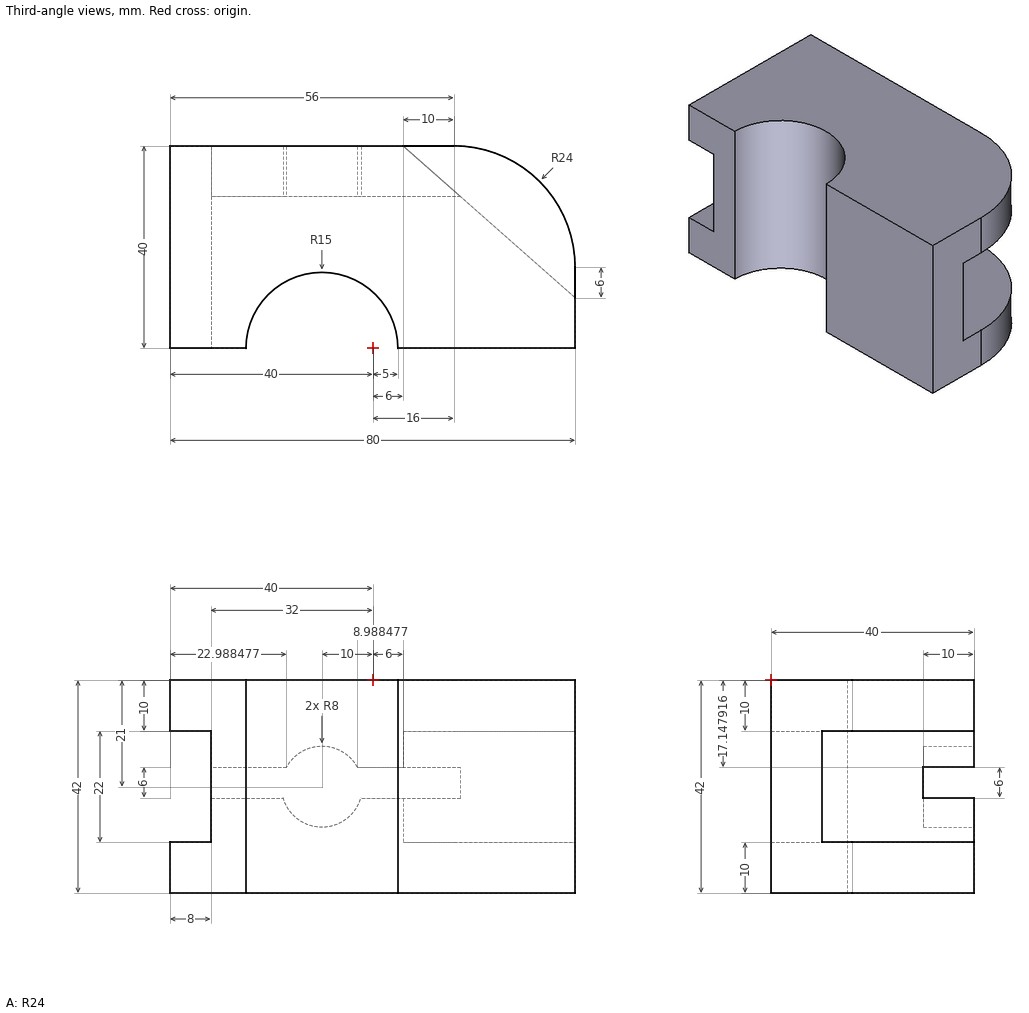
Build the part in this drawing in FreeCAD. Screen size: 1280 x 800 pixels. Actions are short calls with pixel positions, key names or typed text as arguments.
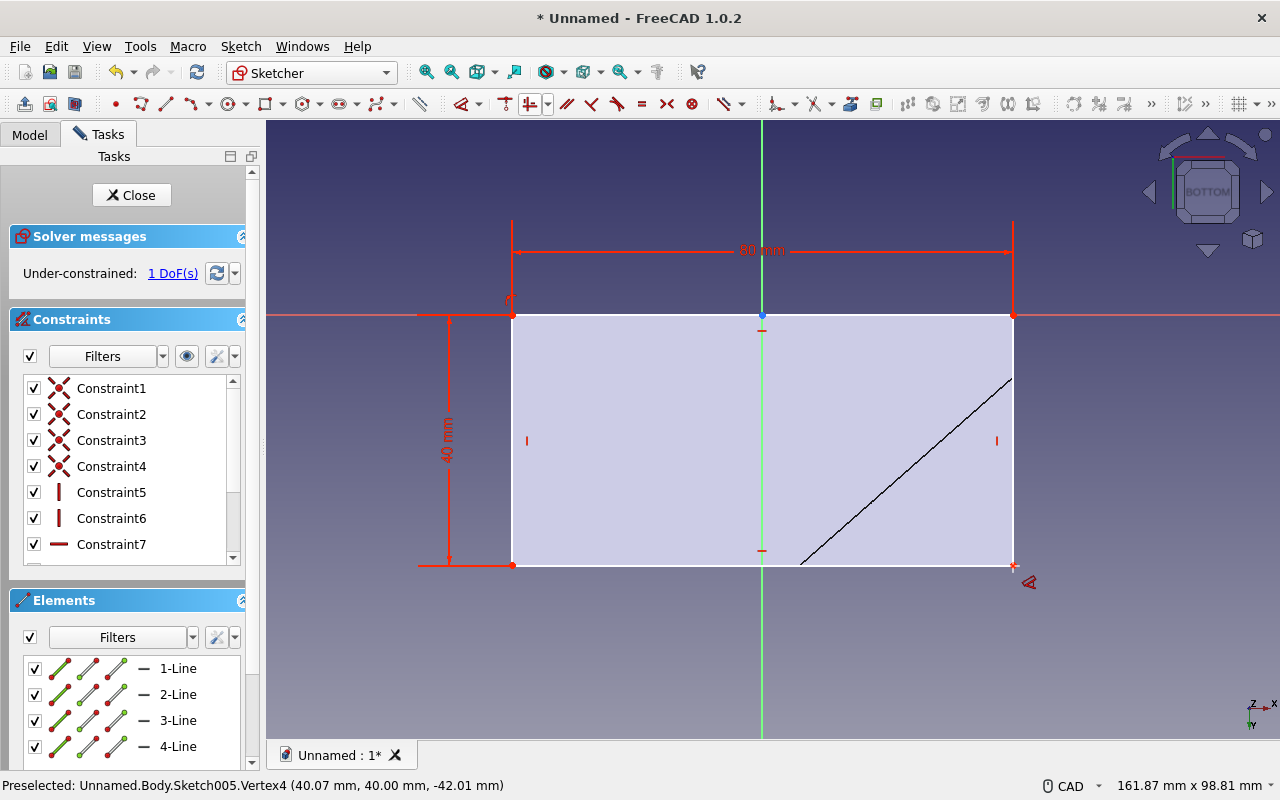
click(512, 315)
click(637, 281)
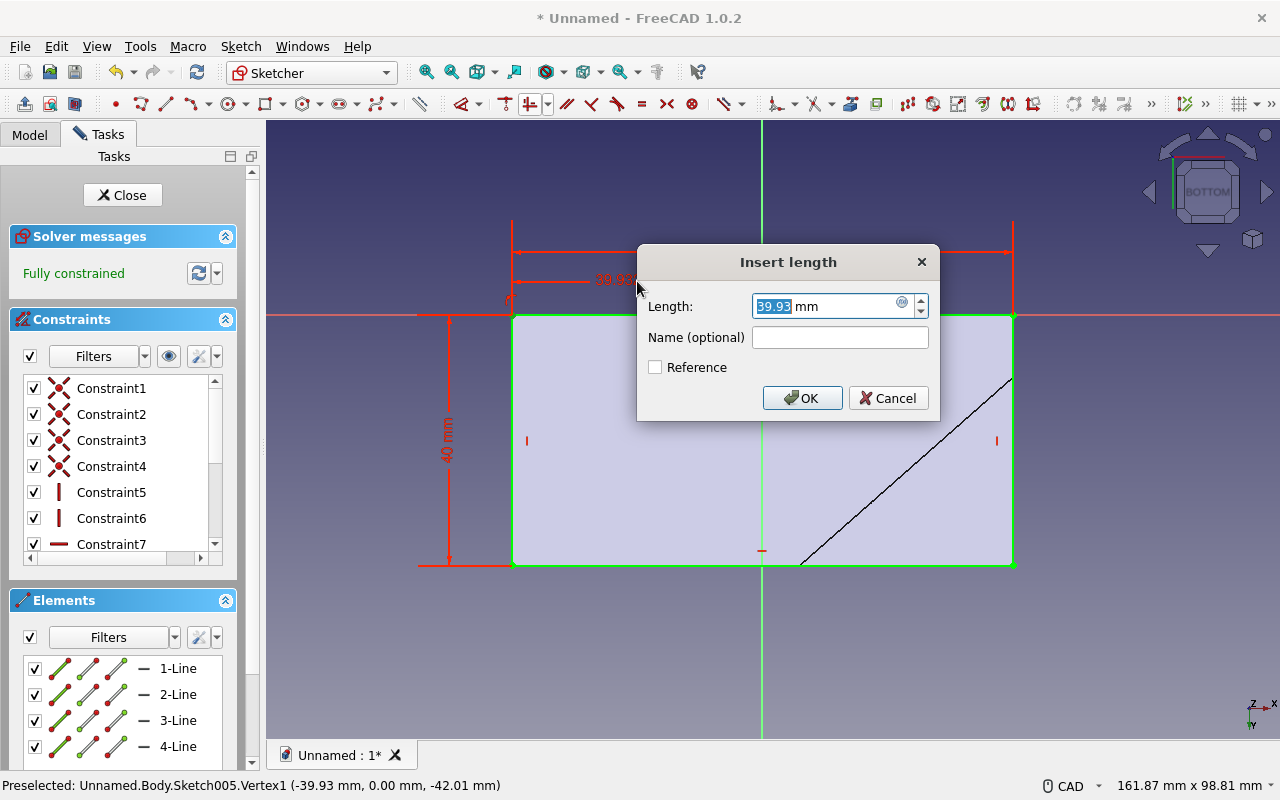
text(40)
key(Return)
key(Escape)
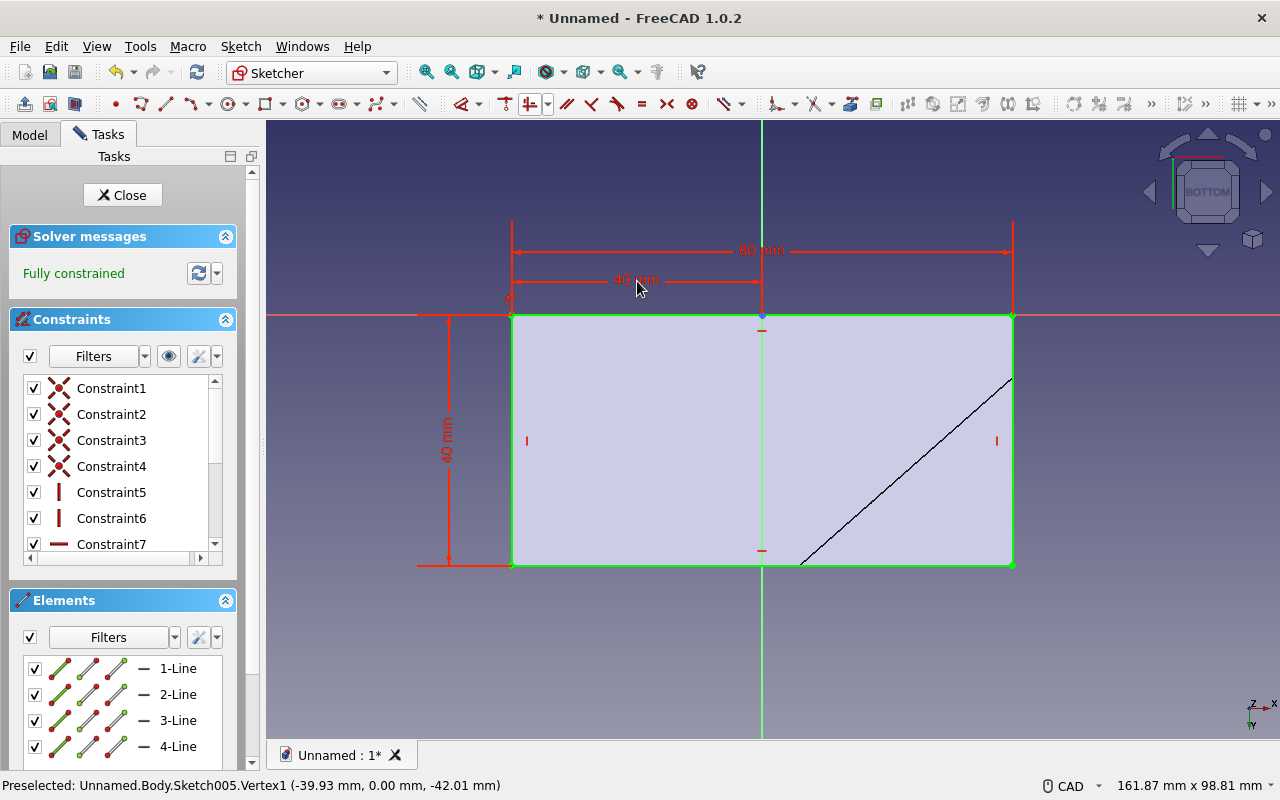
click(123, 195)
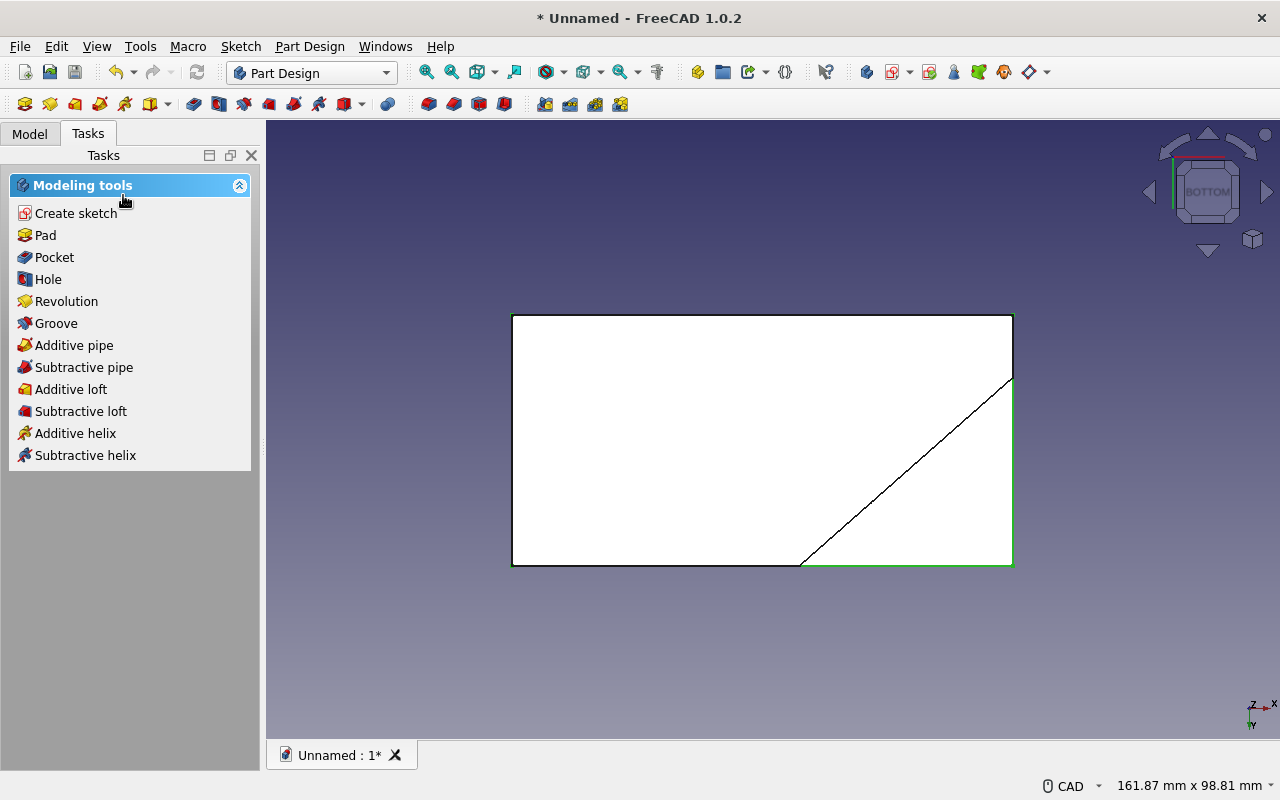
click(25, 104)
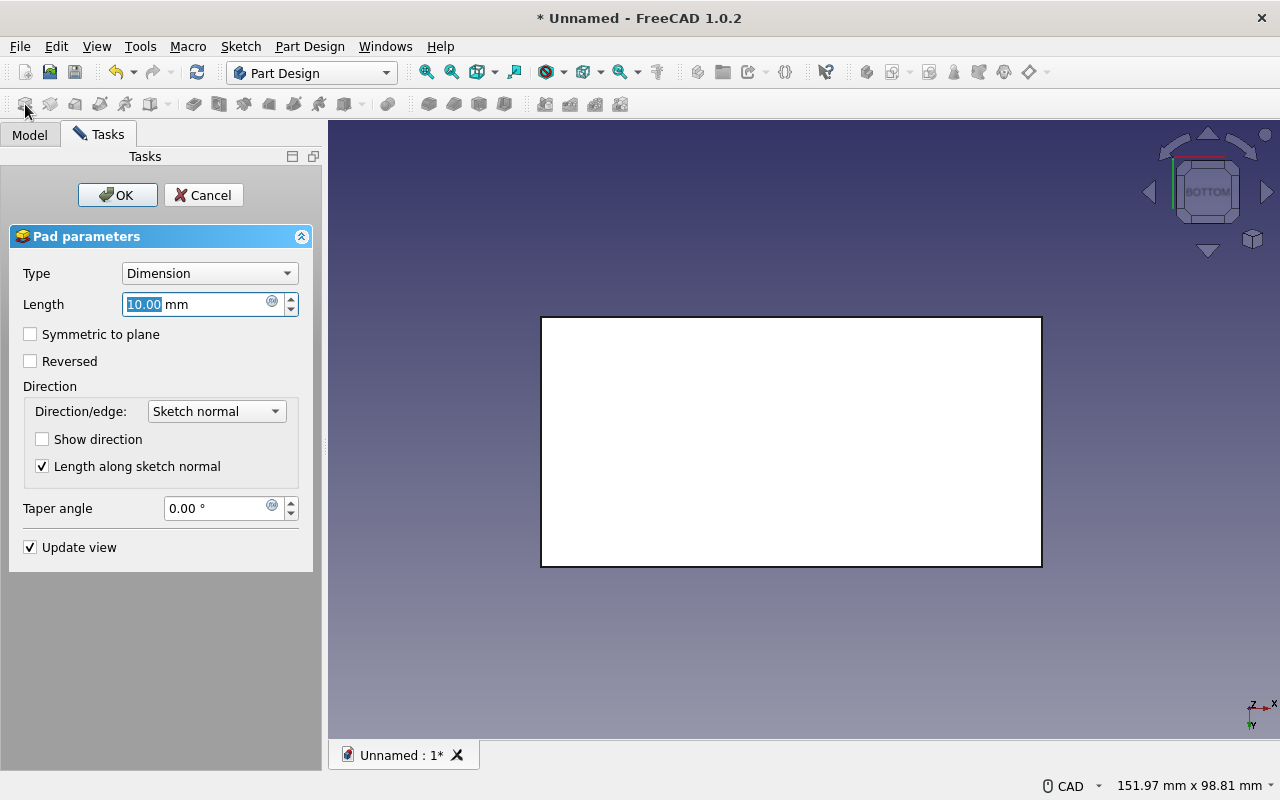
text(10)
key(Tab)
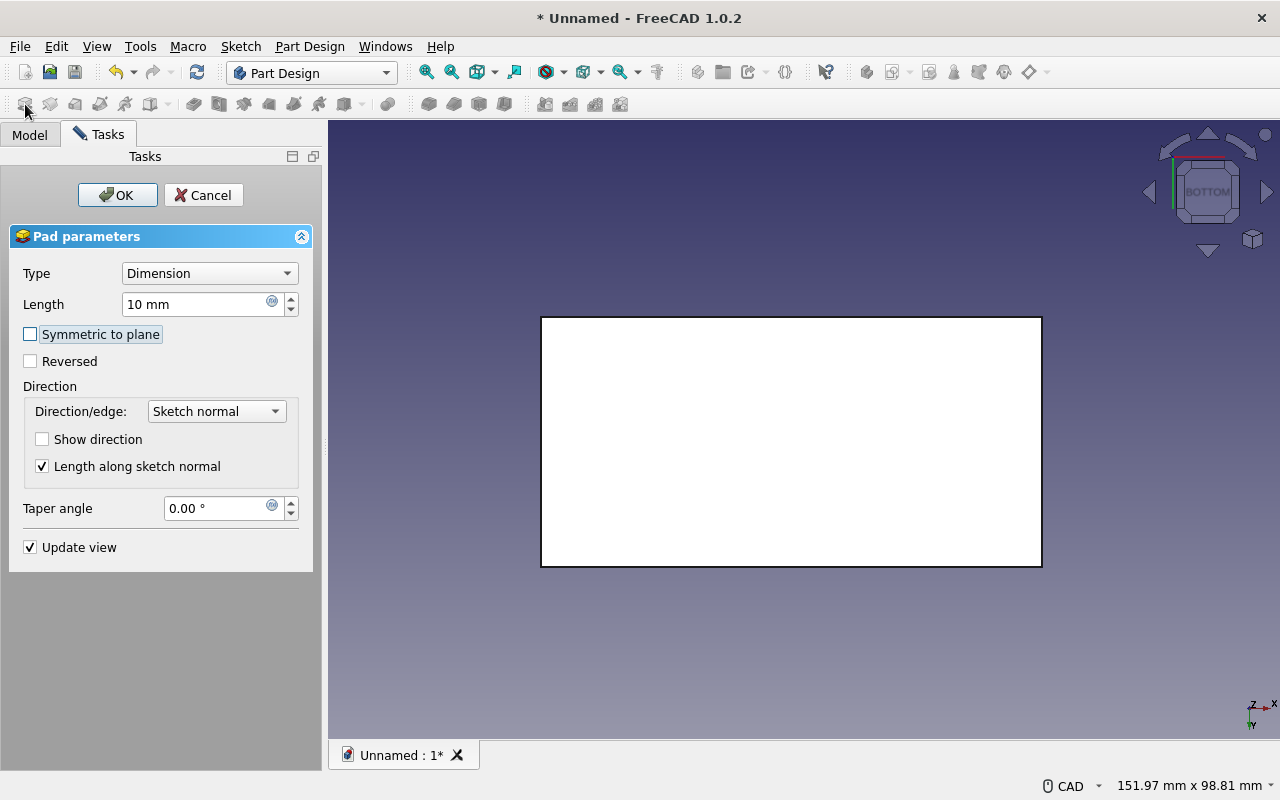
click(31, 361)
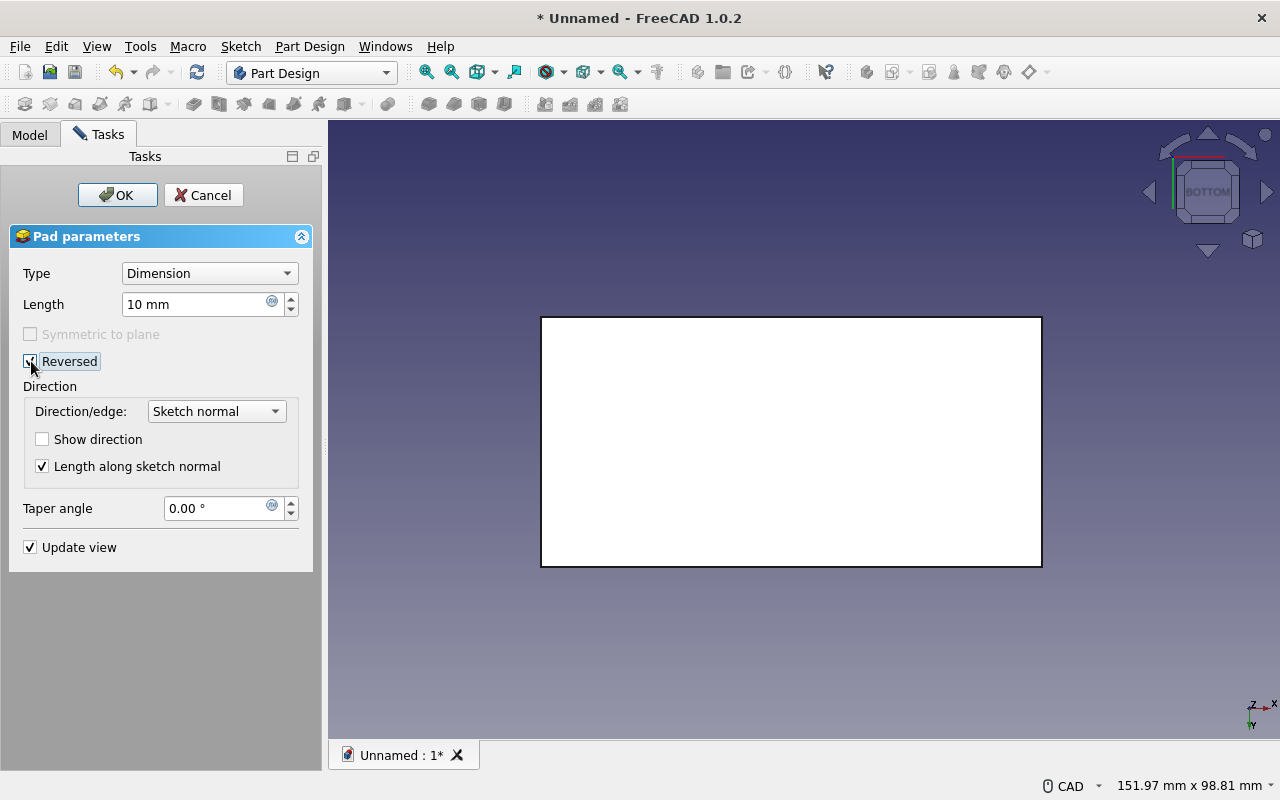
click(118, 195)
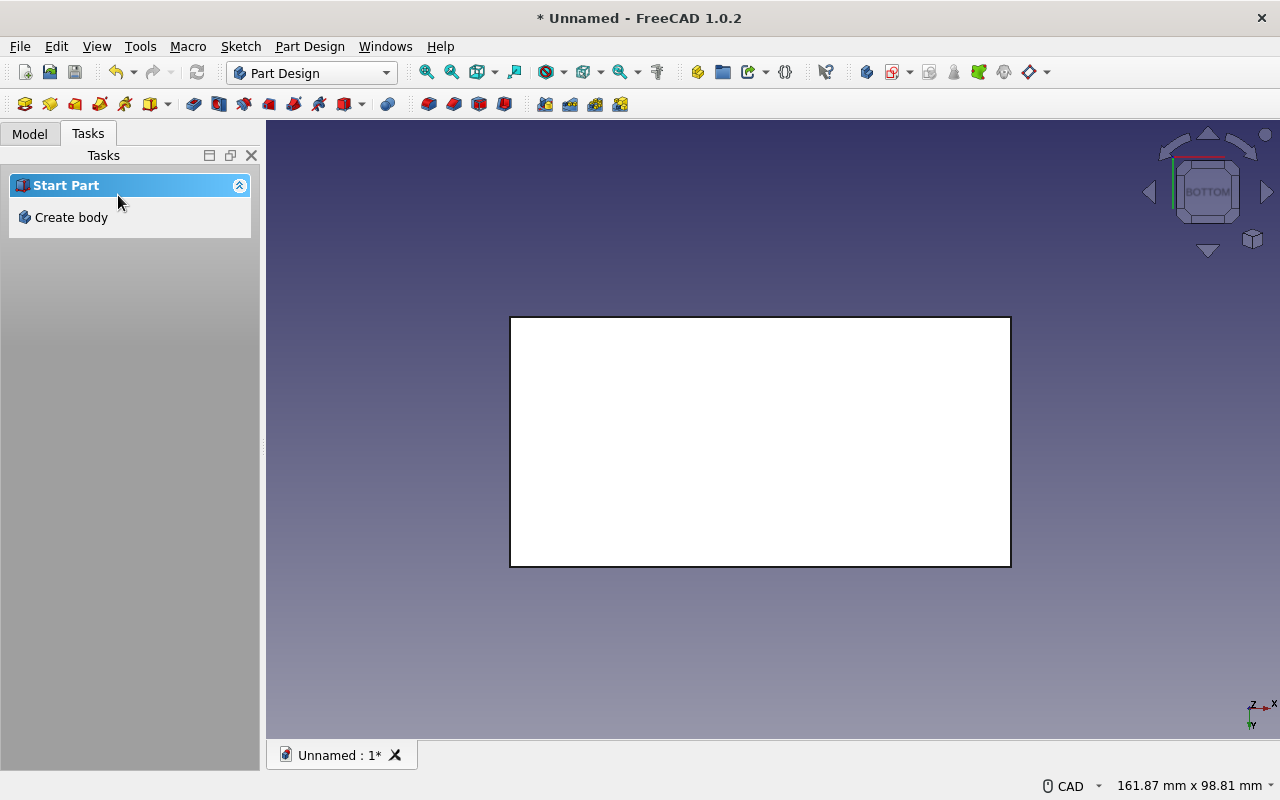
key(0)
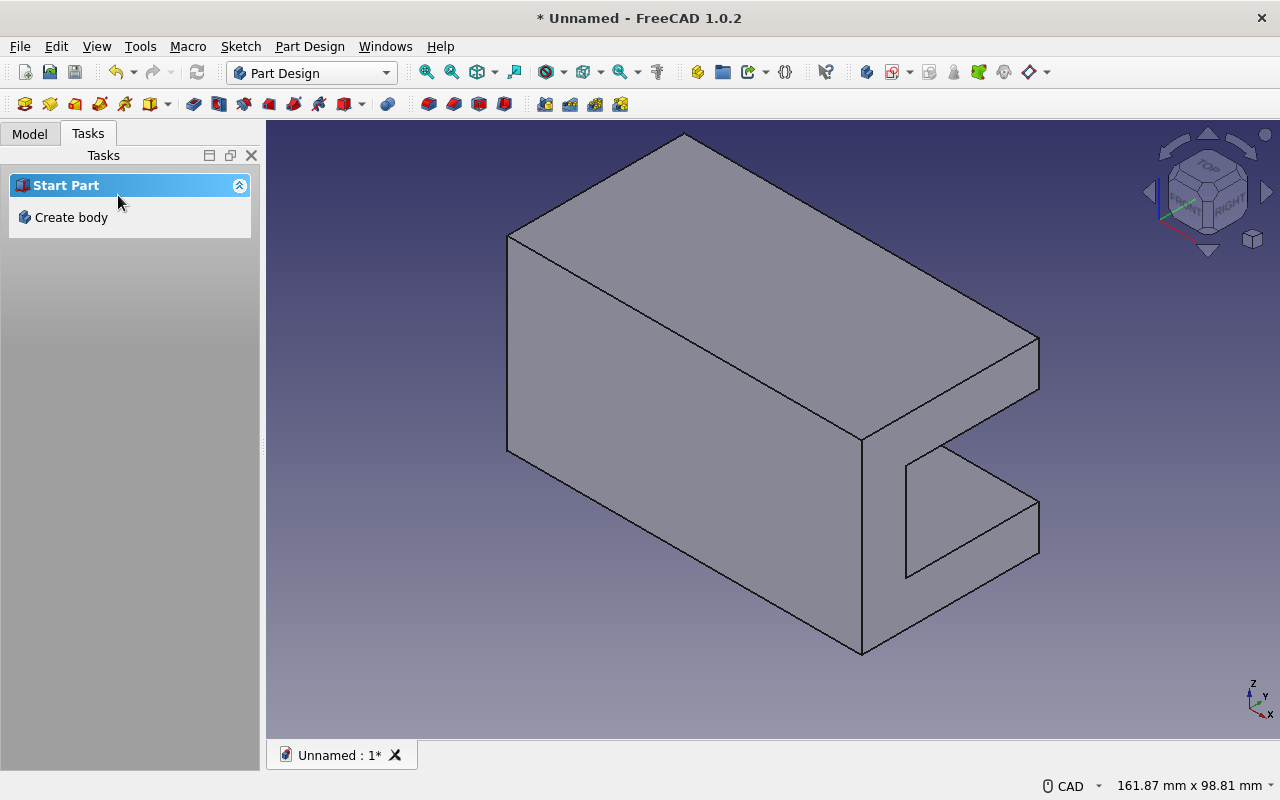
key(2)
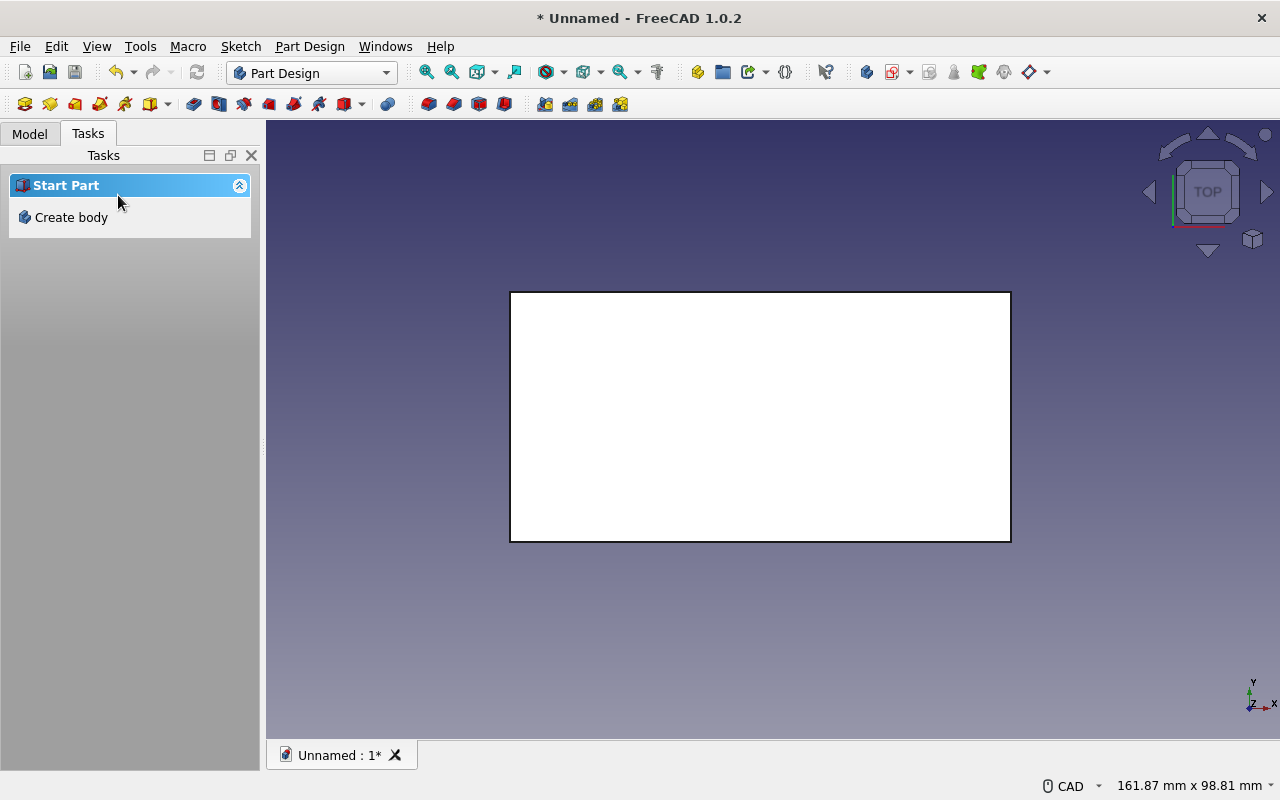
key(1)